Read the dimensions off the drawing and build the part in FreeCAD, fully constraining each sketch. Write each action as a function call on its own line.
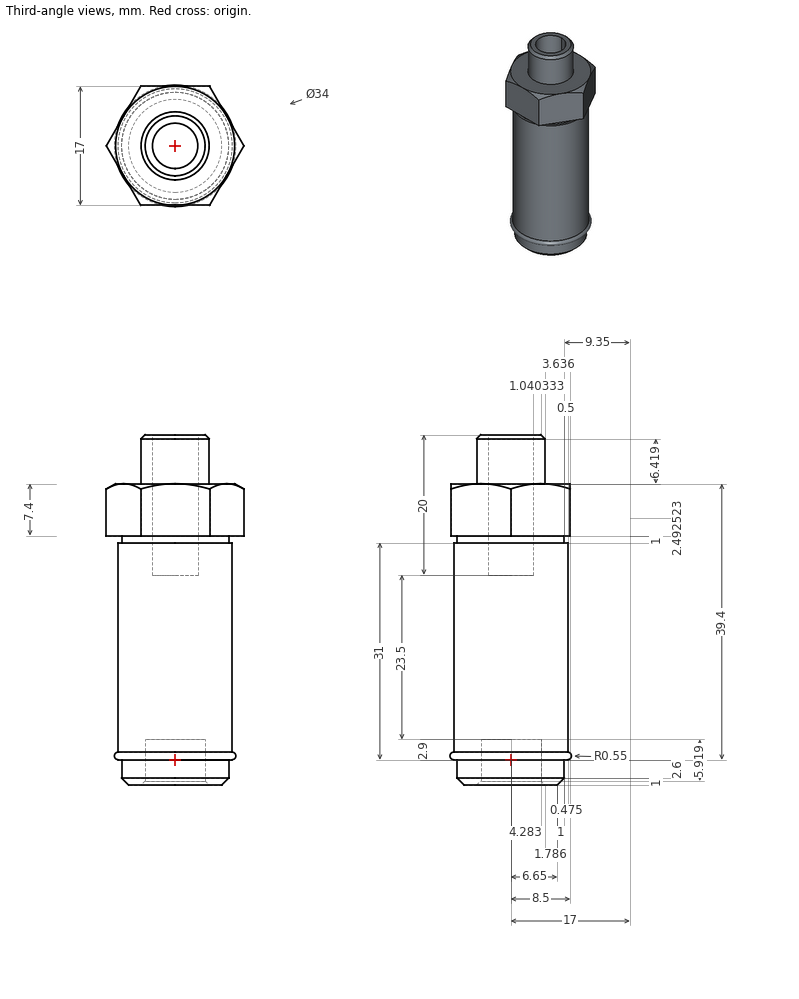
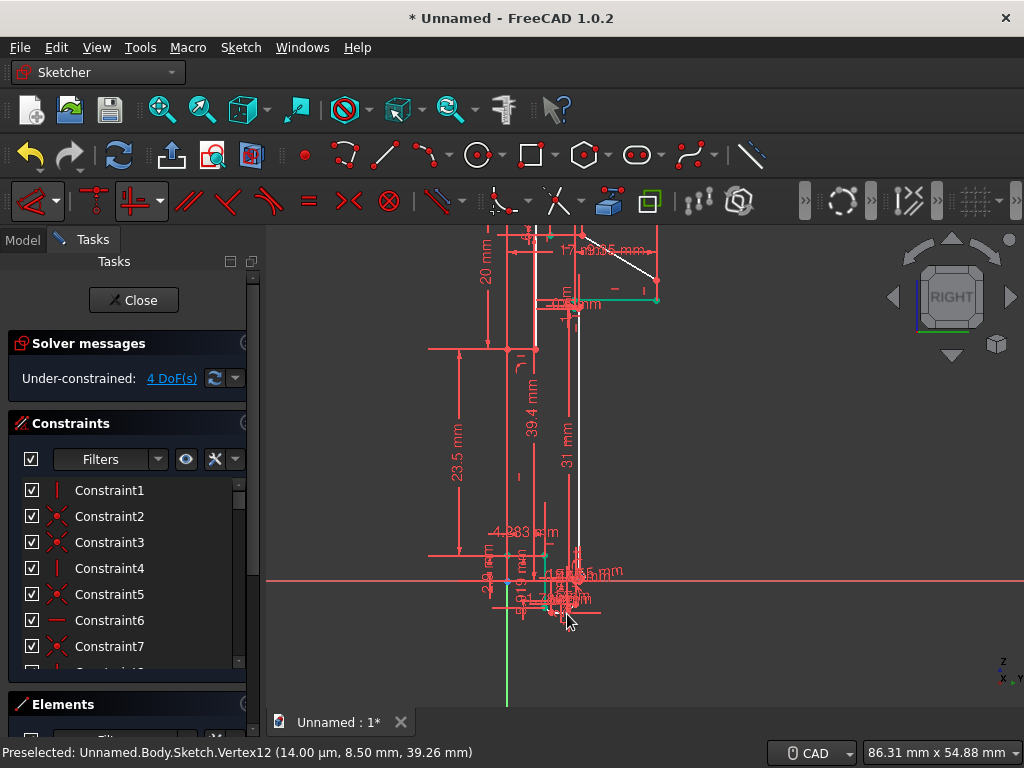
click(567, 613)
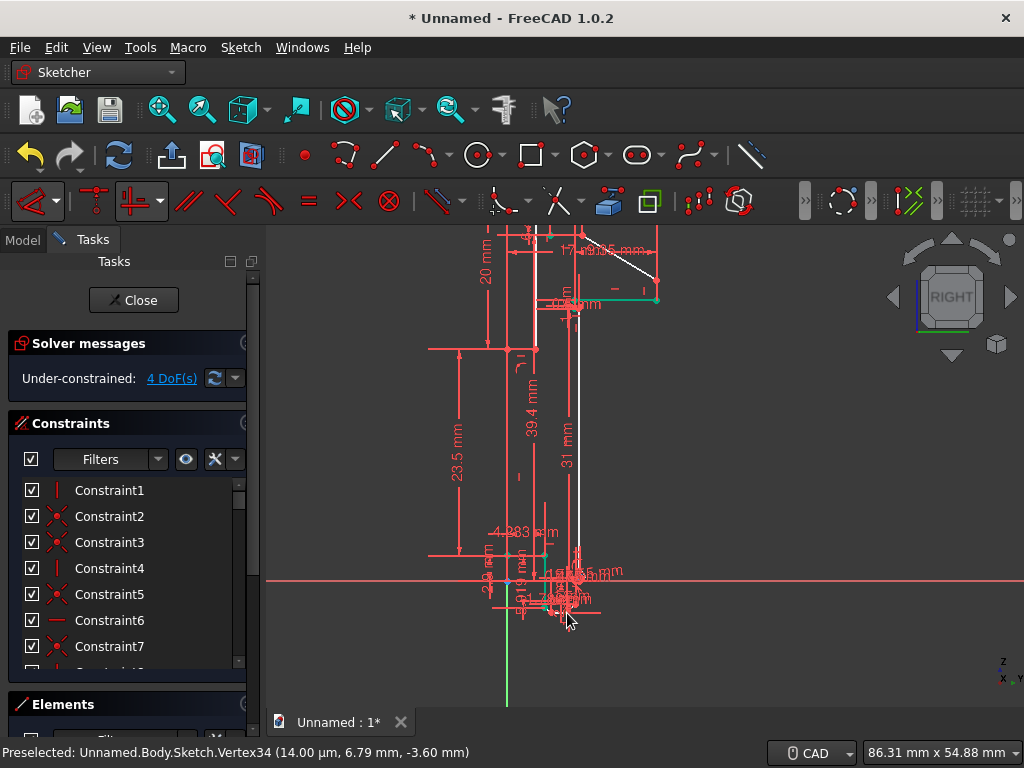
key(l)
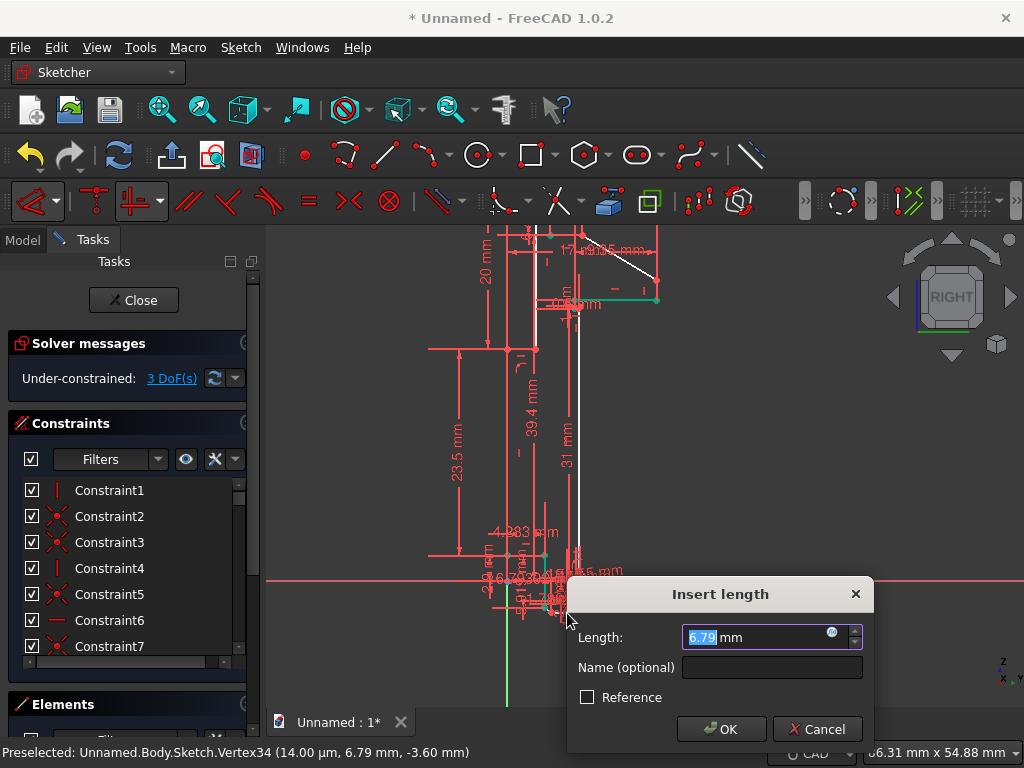
text(6.65)
key(Return)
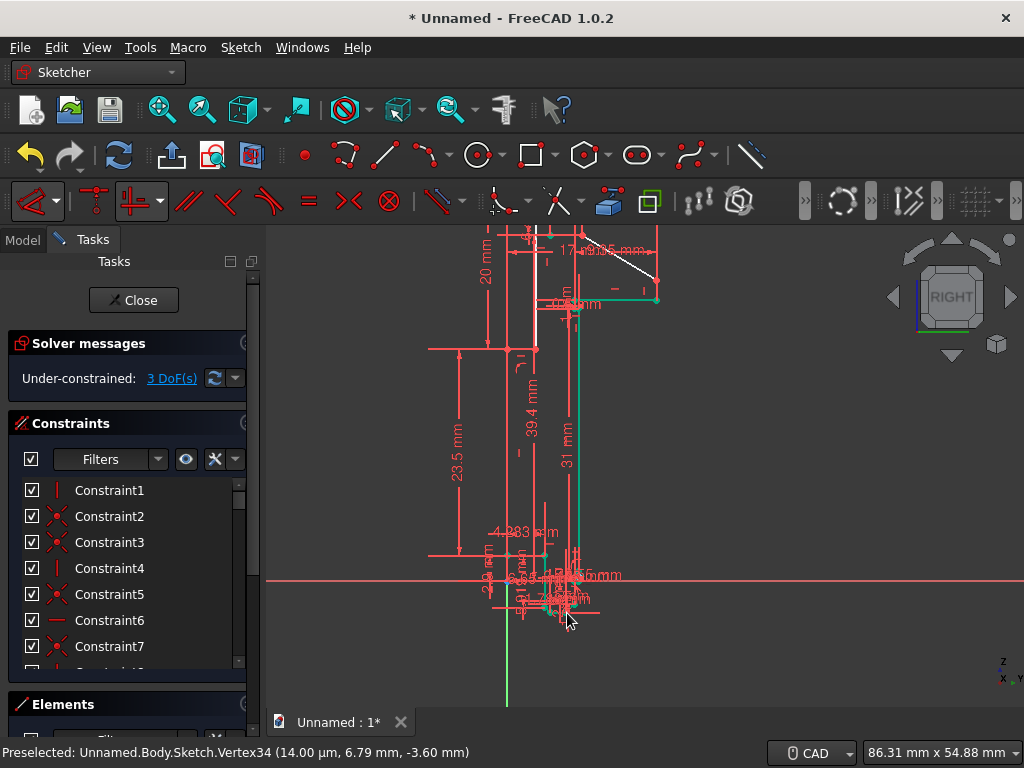
scroll(565, 614, down, 2)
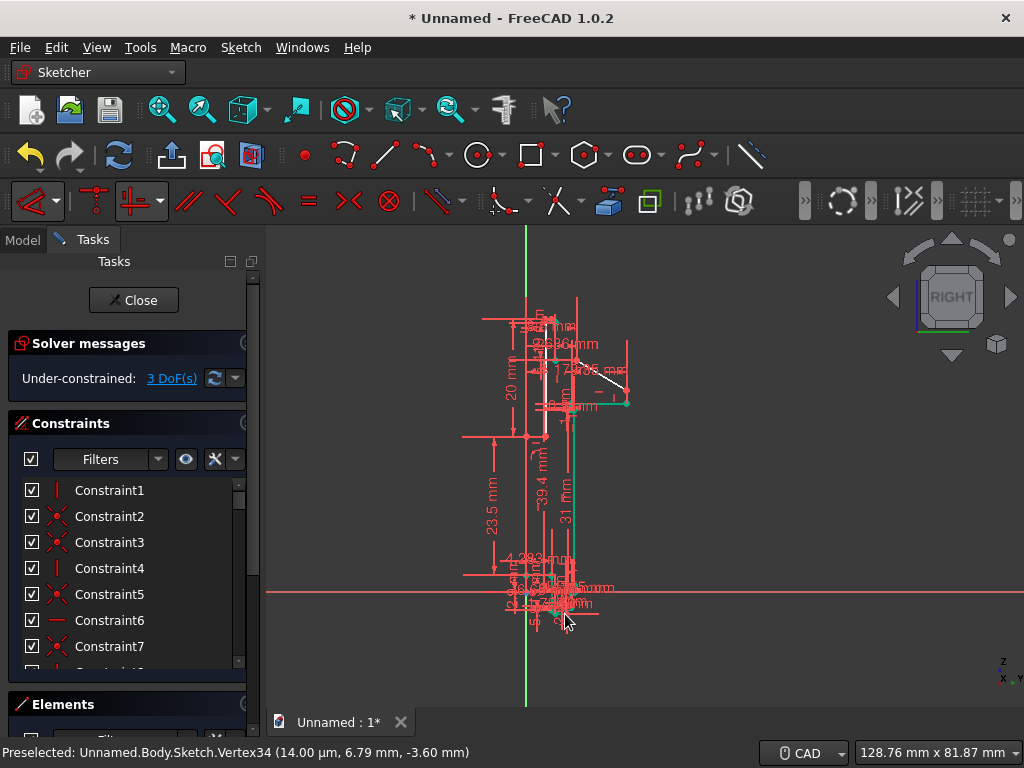
scroll(552, 319, up, 5)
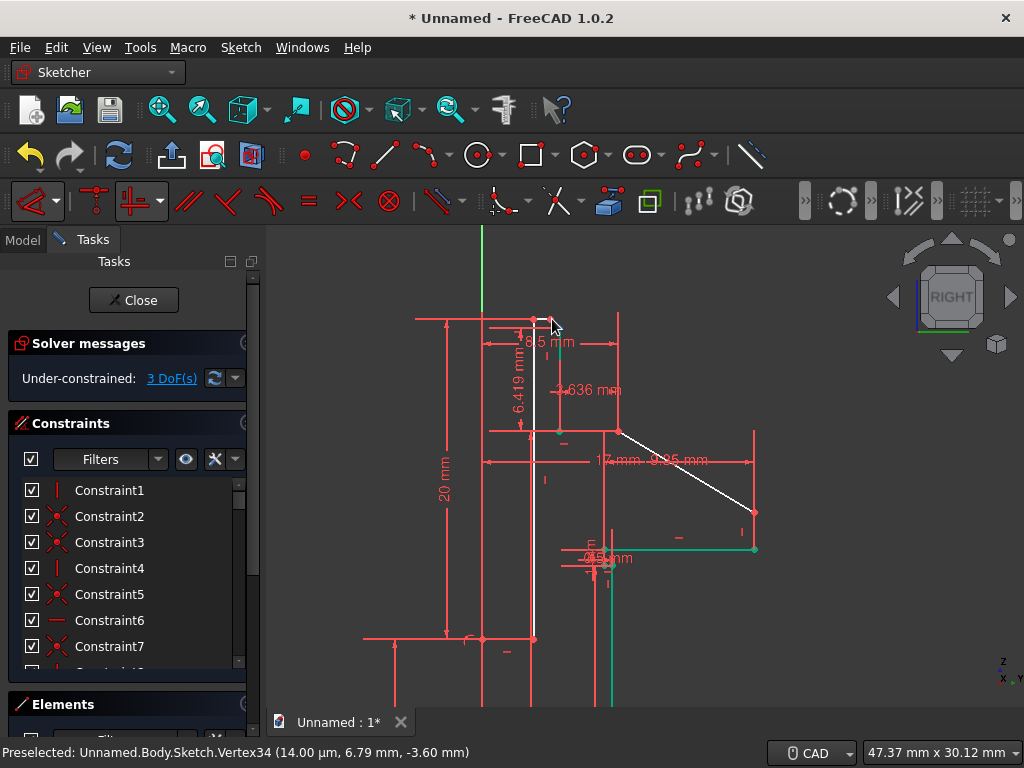
click(550, 319)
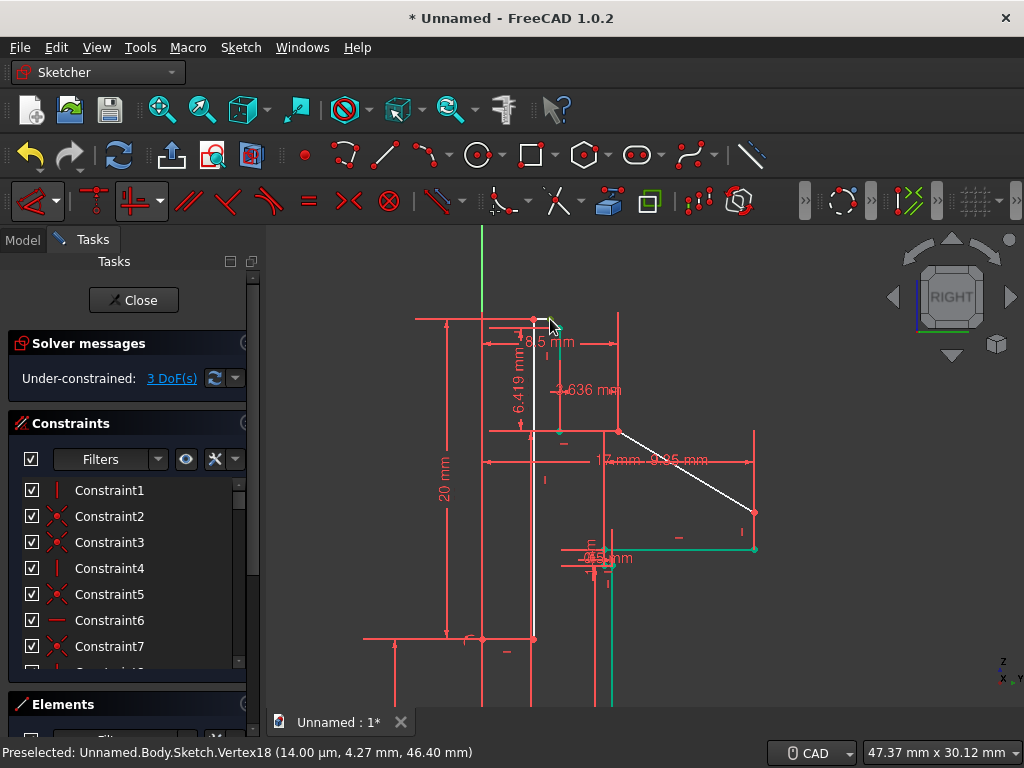
key(l)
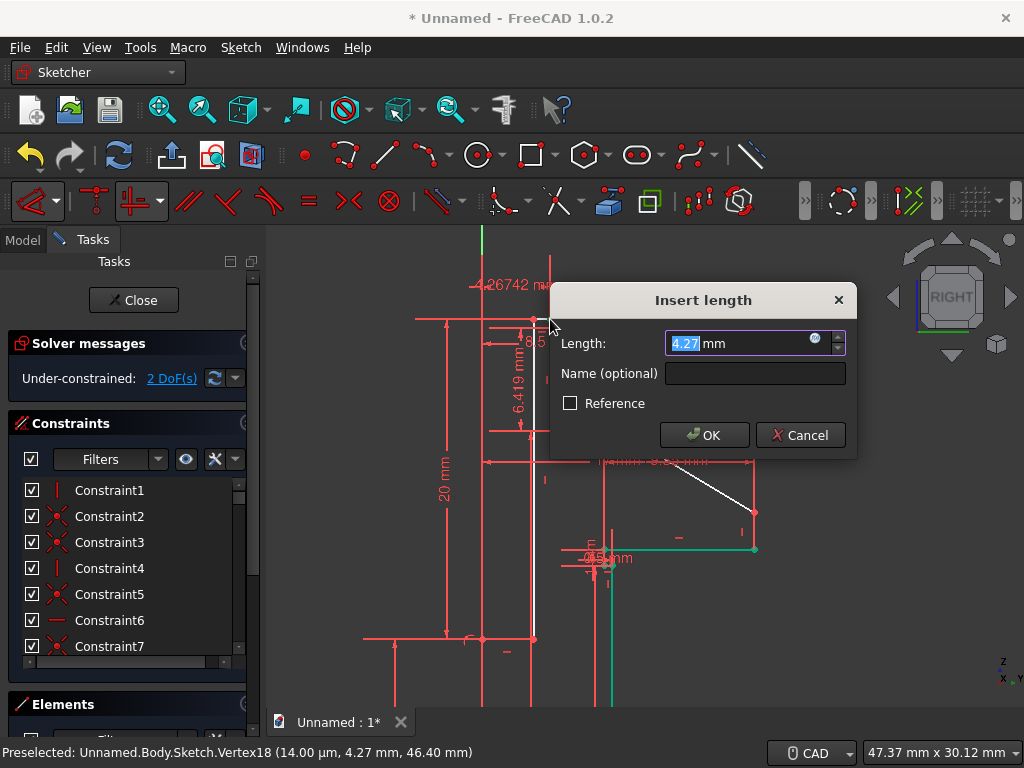
text(4.283)
key(Return)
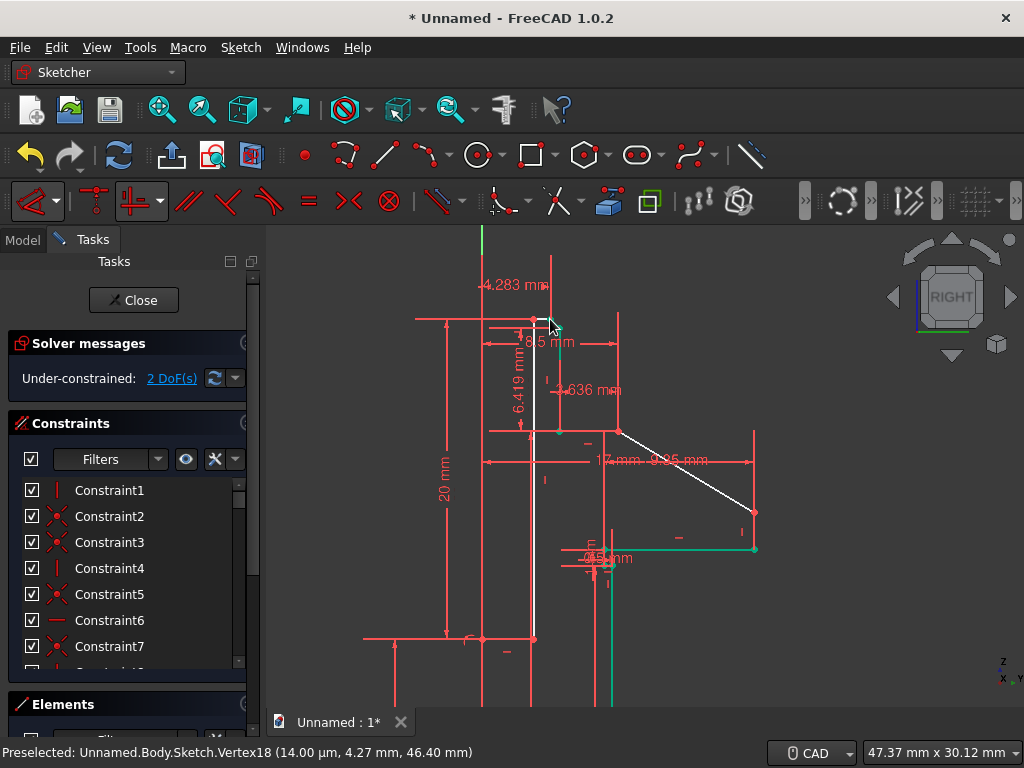
scroll(754, 538, up, 2)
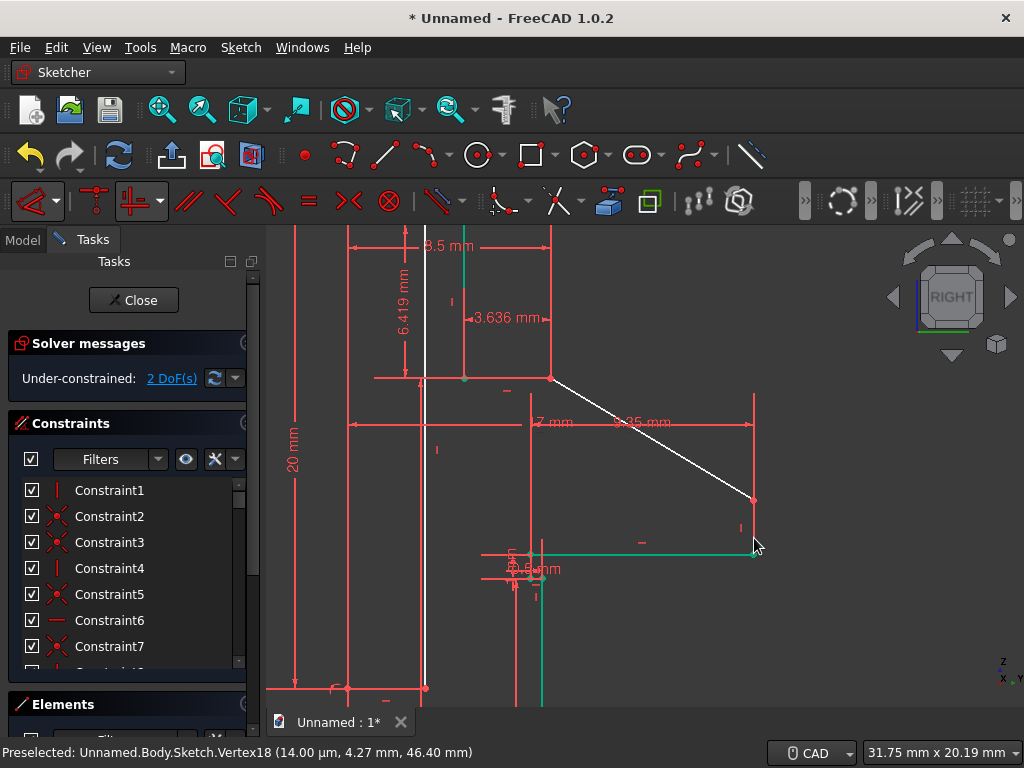
click(754, 538)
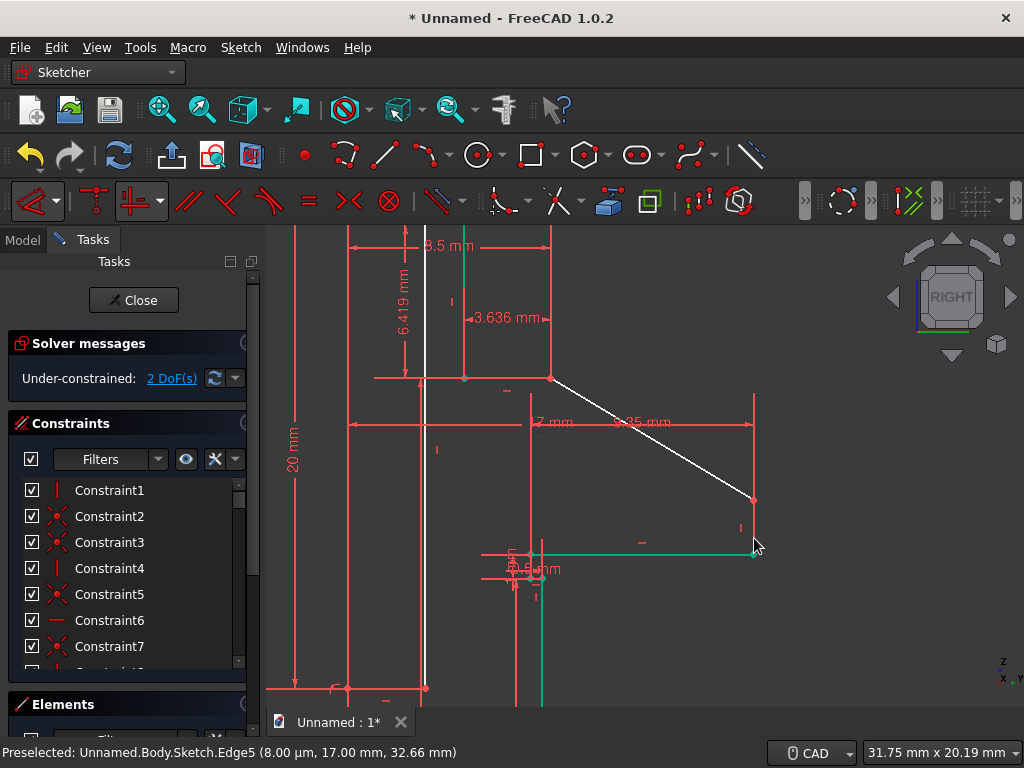
key(i)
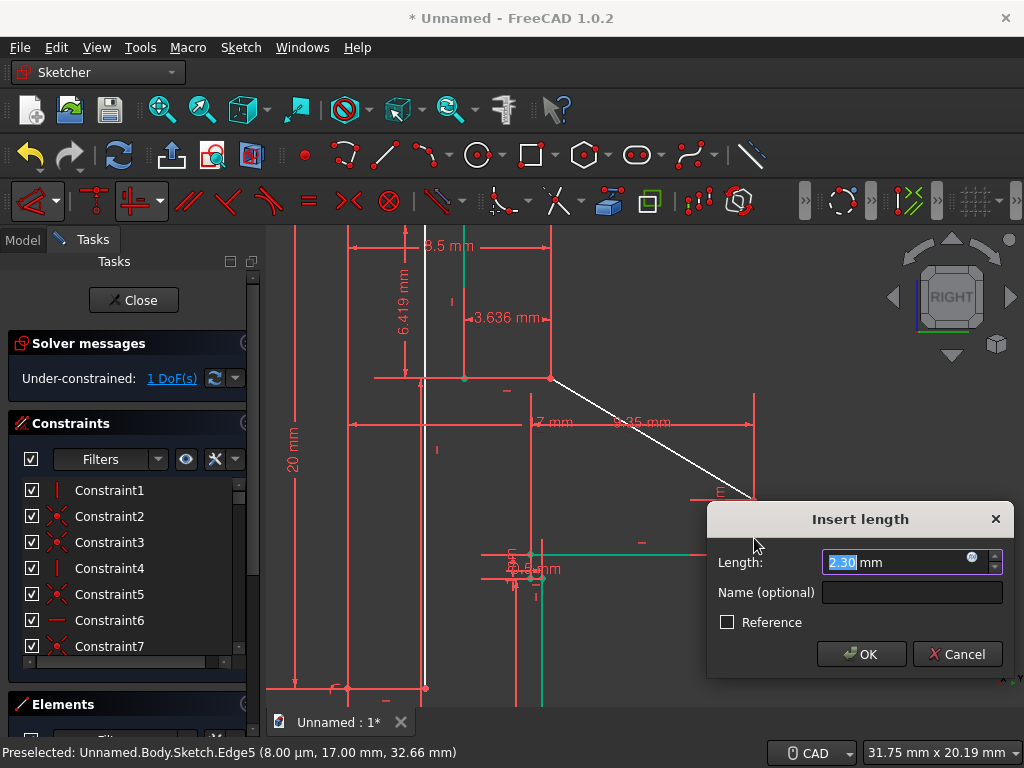
text(2.492523)
key(Return)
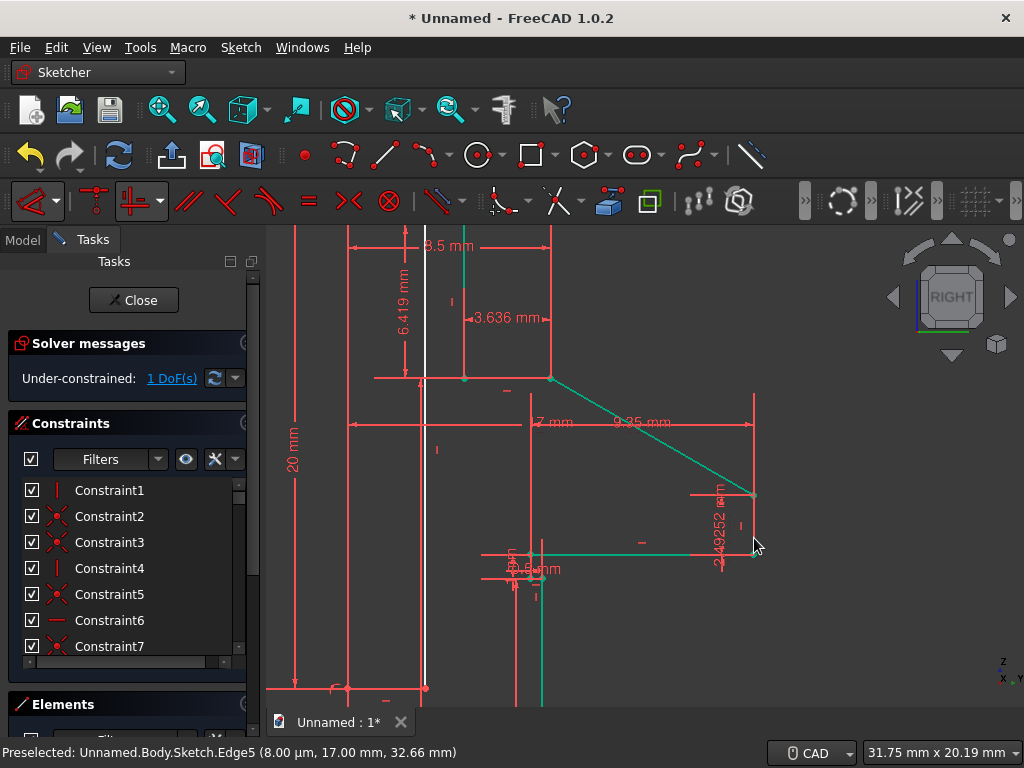
scroll(585, 354, down, 7)